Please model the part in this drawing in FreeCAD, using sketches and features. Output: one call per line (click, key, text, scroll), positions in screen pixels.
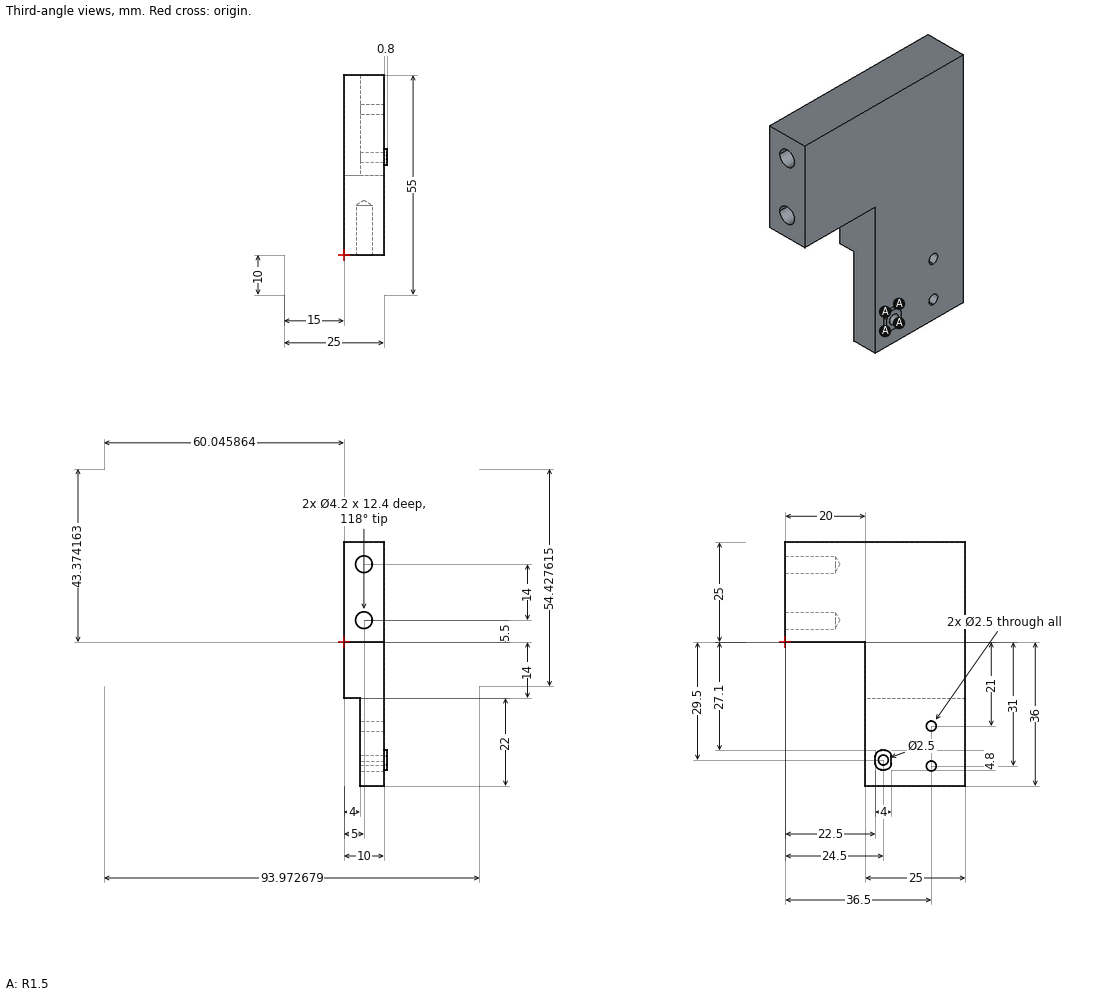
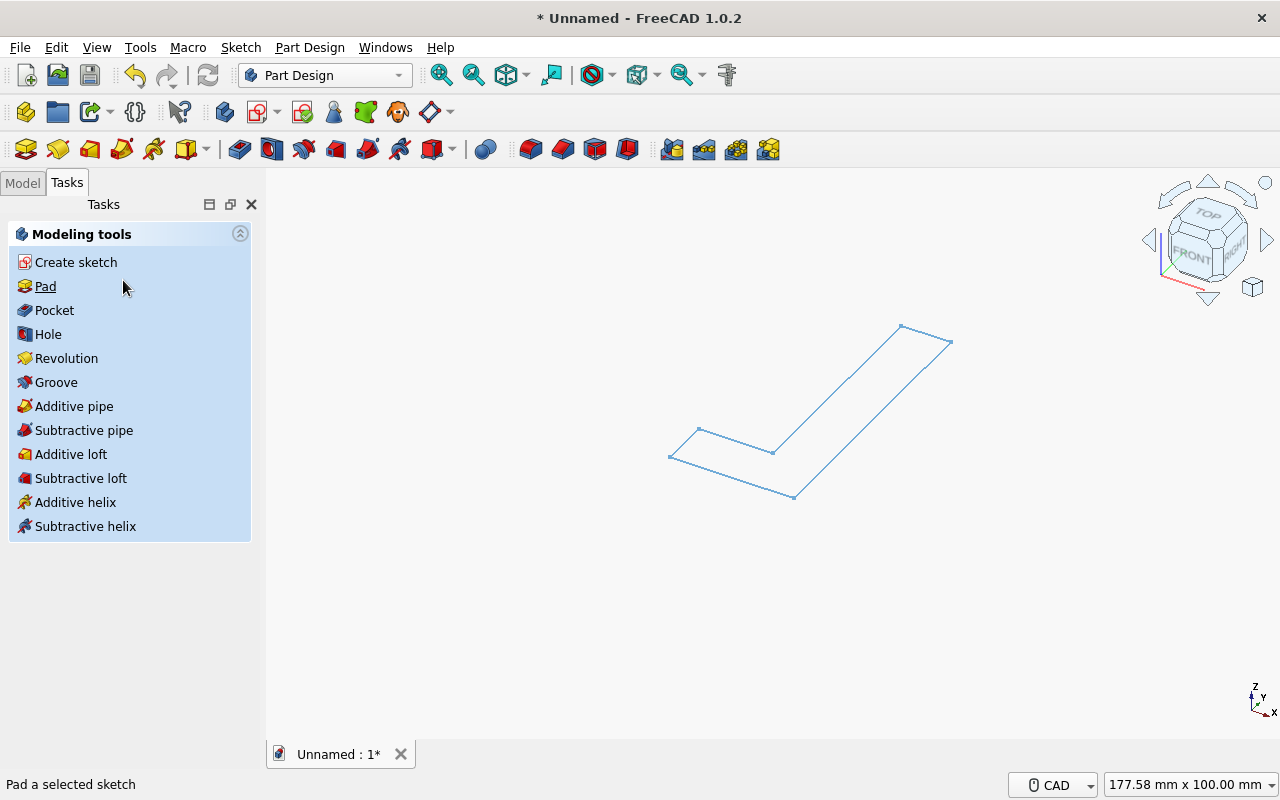
click(26, 150)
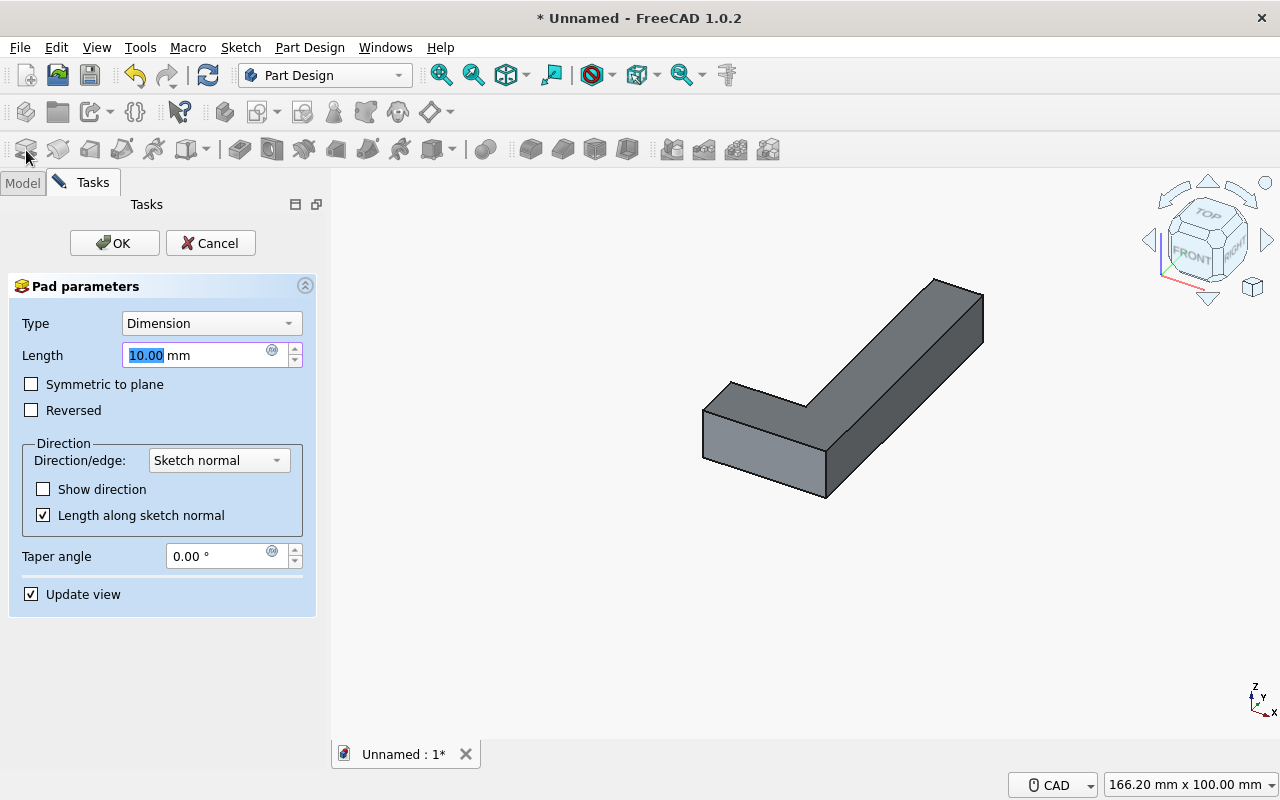
text(25)
key(Tab)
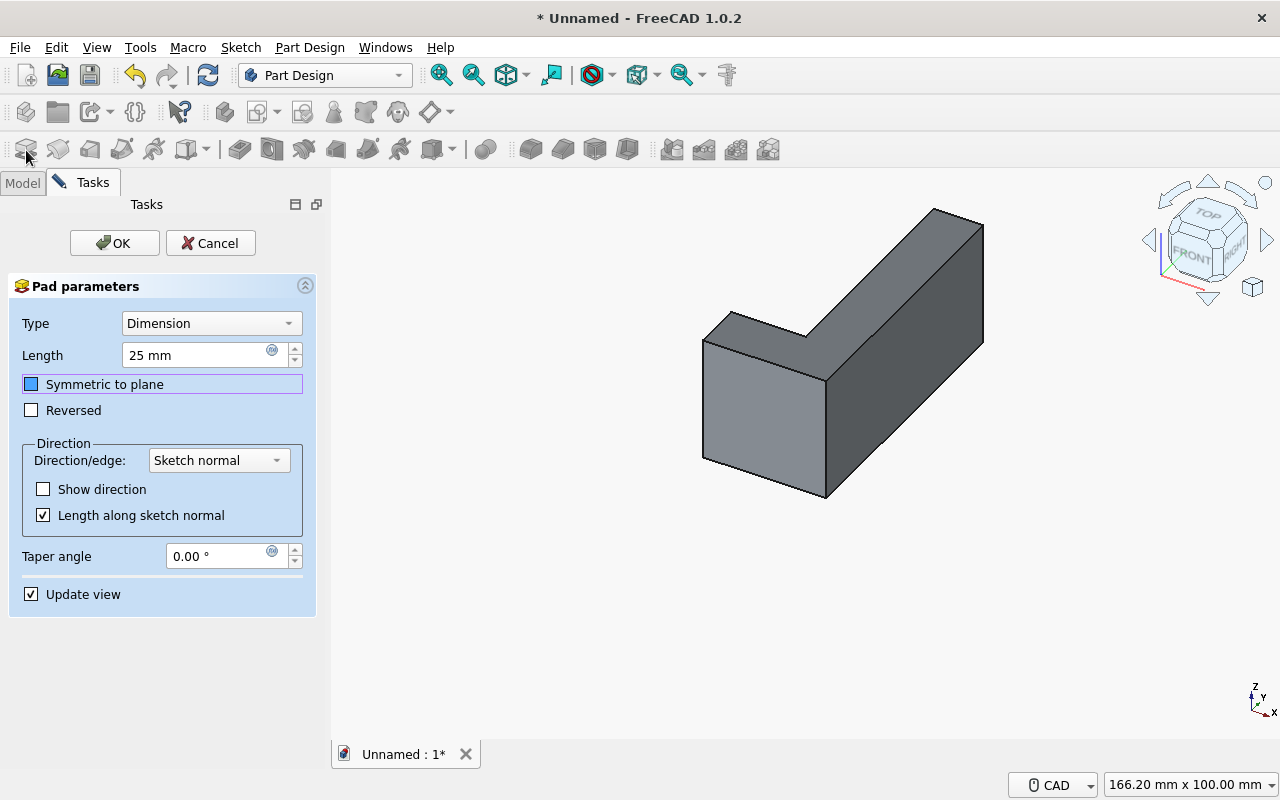
click(115, 243)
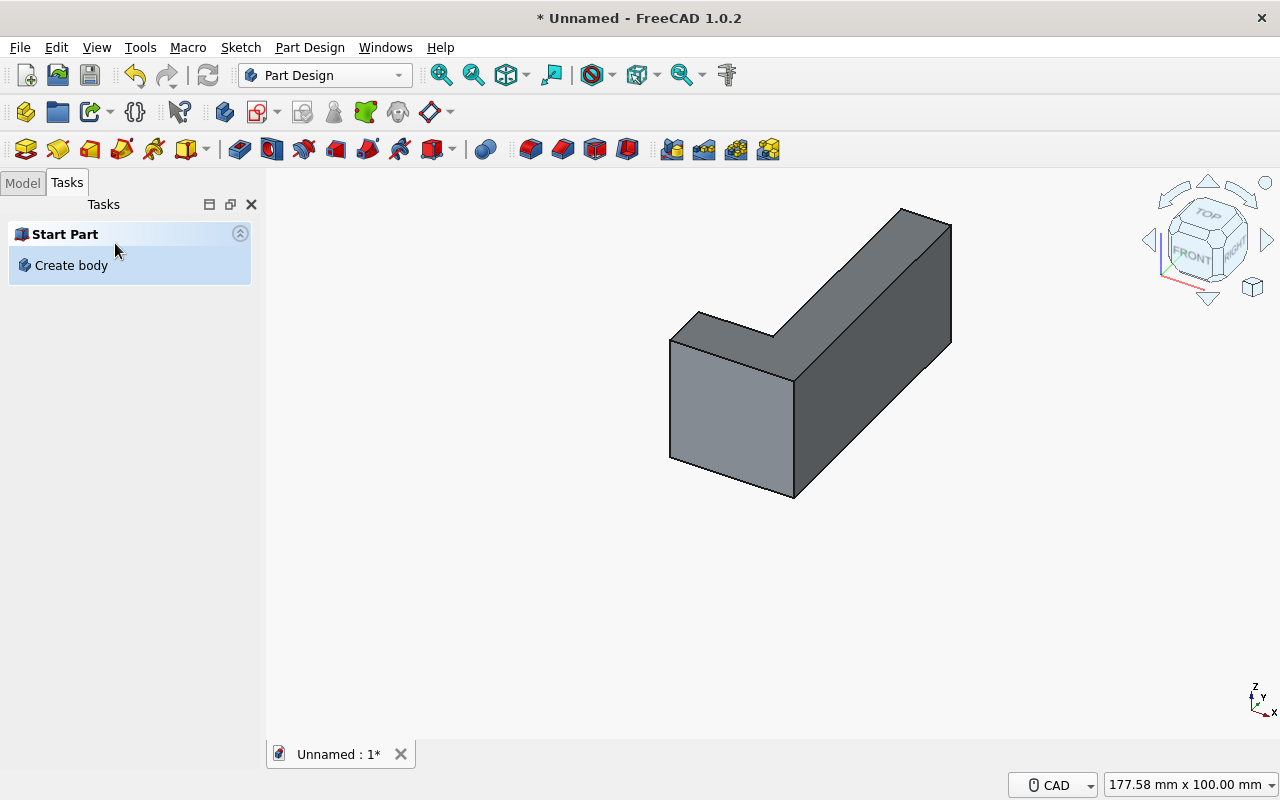
click(258, 112)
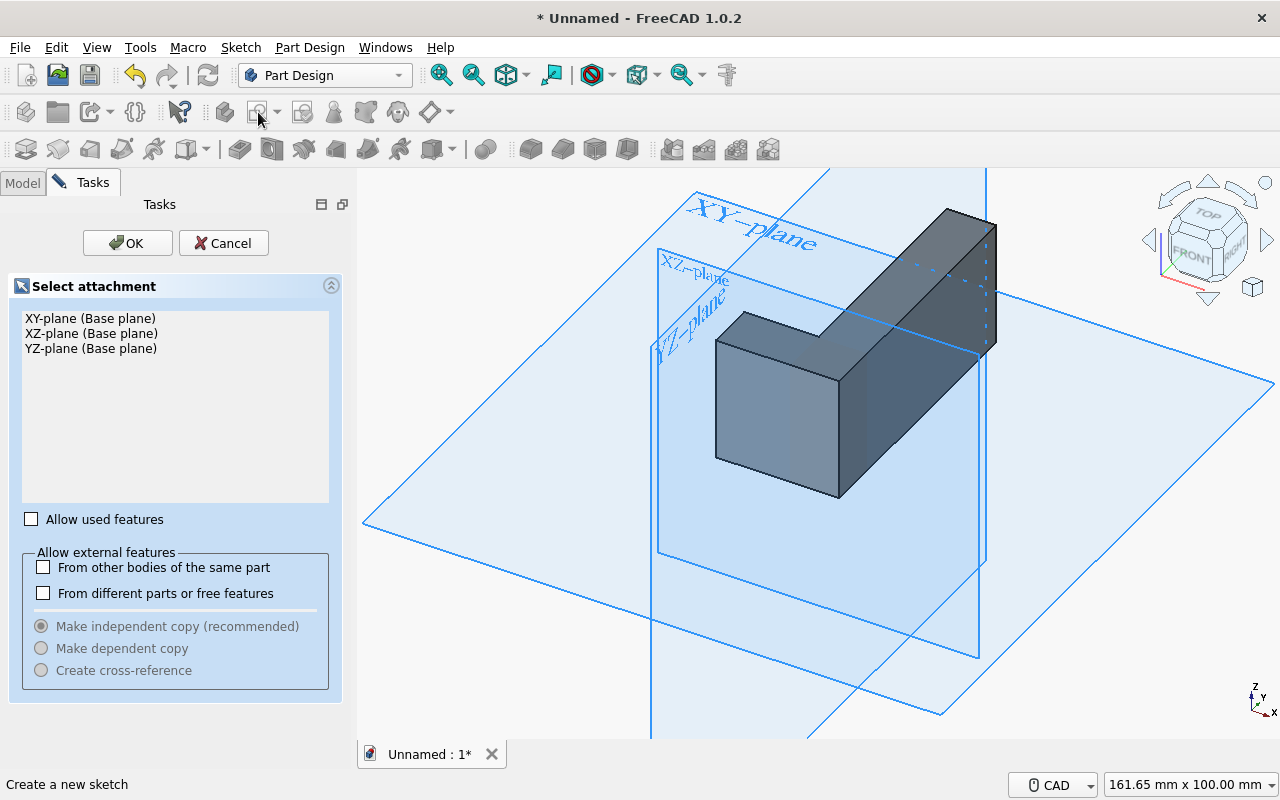
click(82, 348)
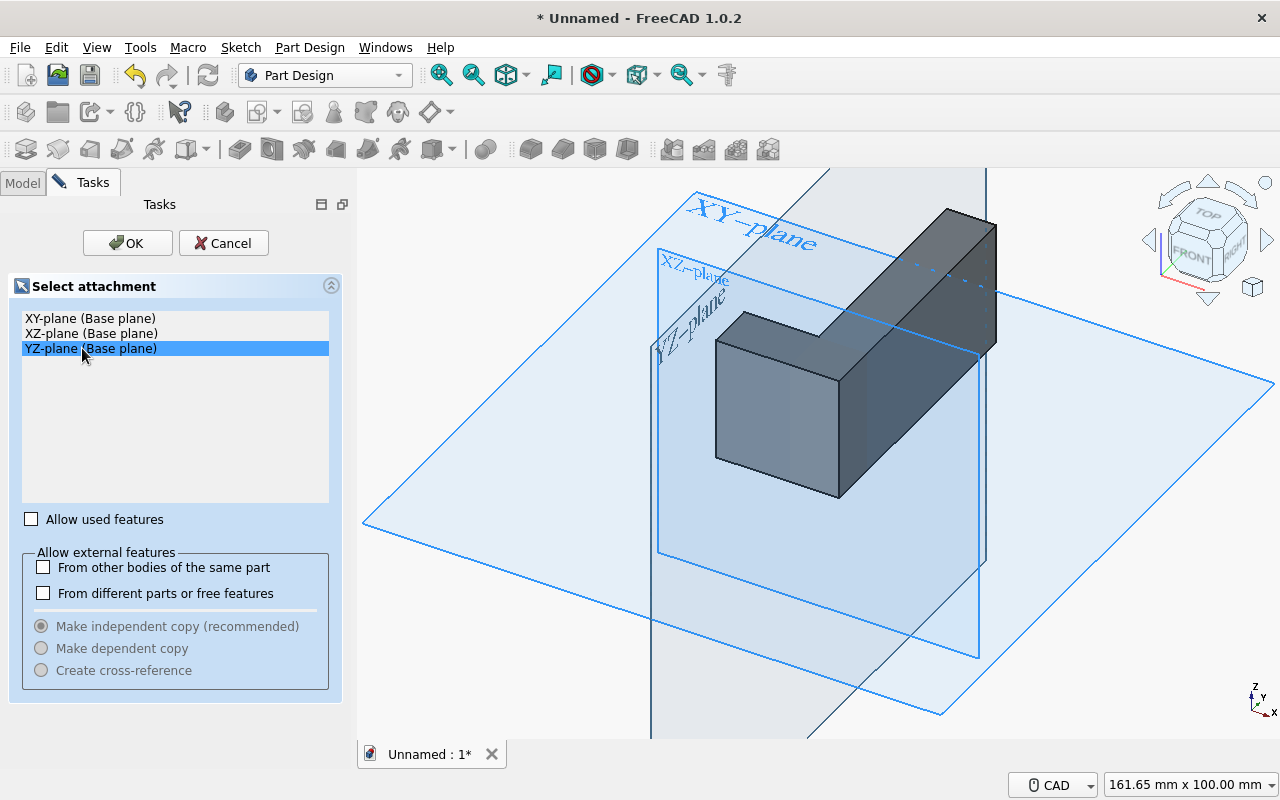
click(128, 243)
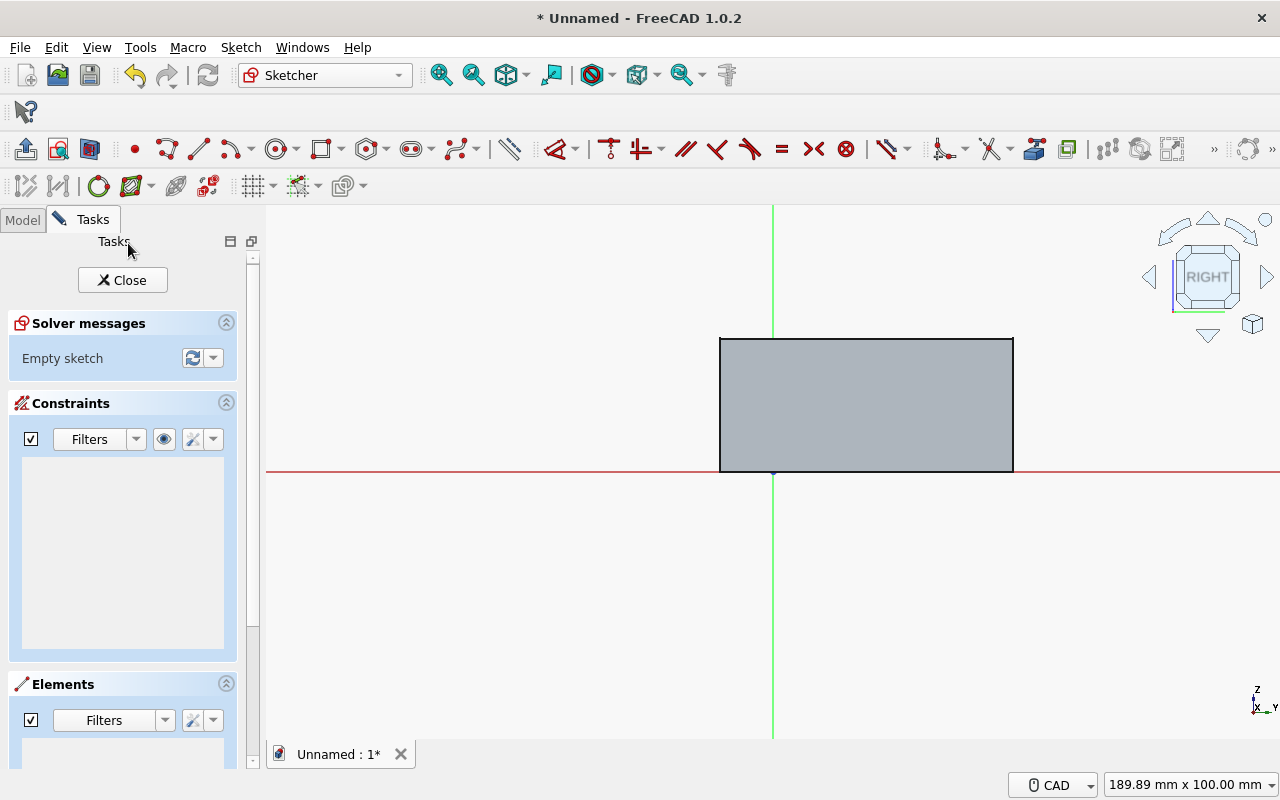
click(90, 150)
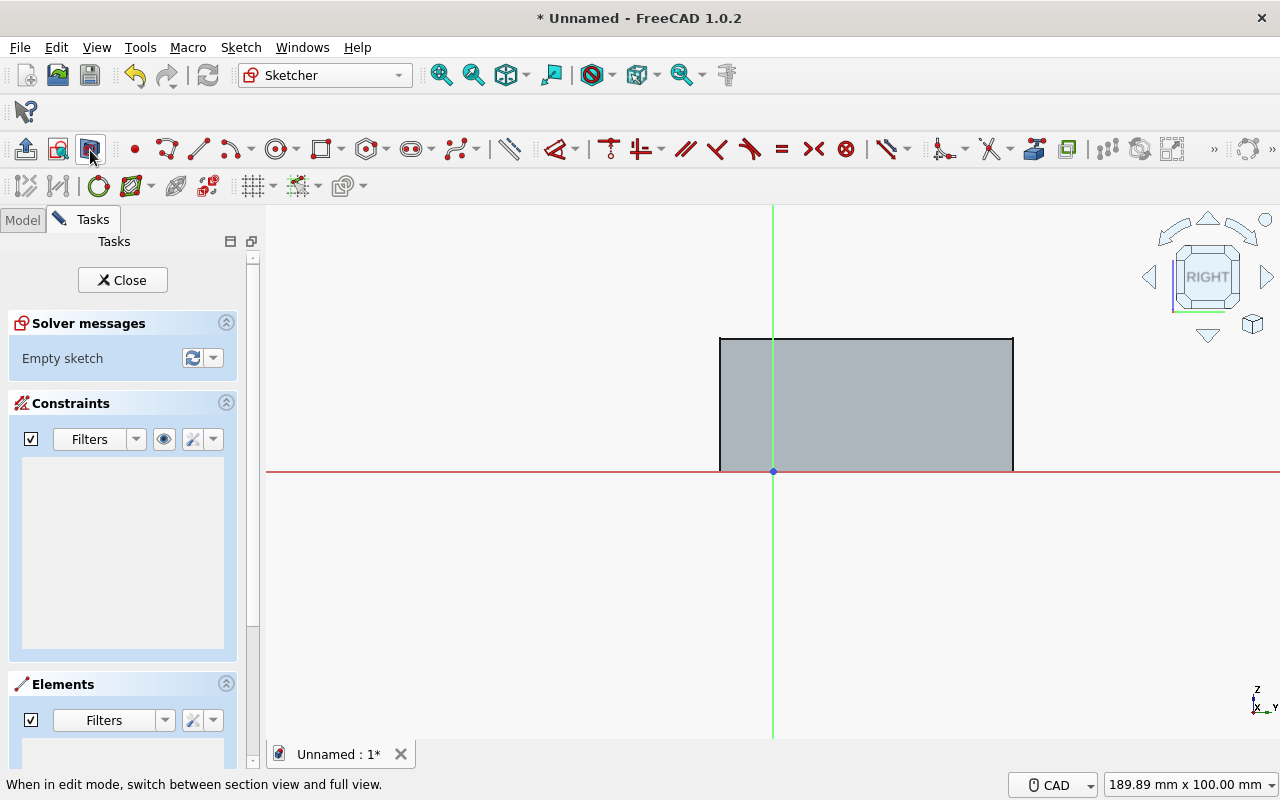
scroll(1115, 685, up, 3)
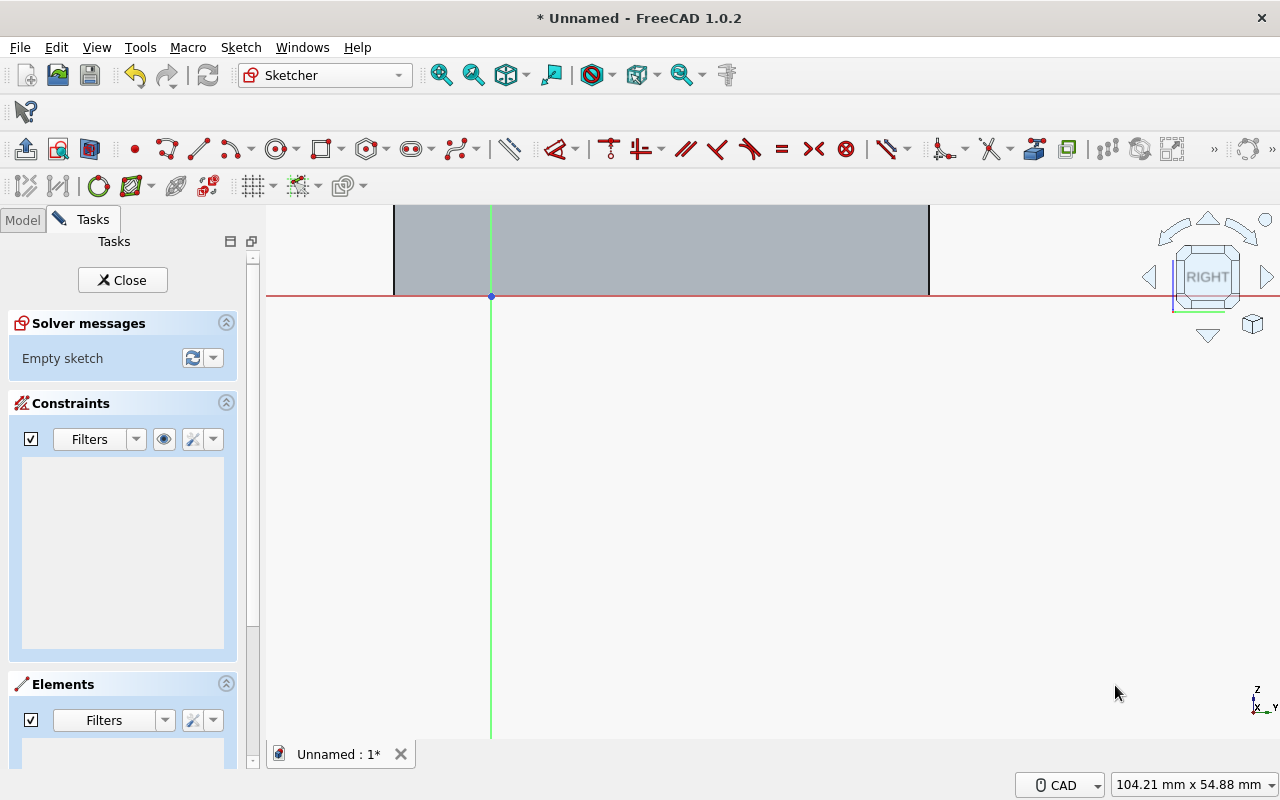
click(322, 150)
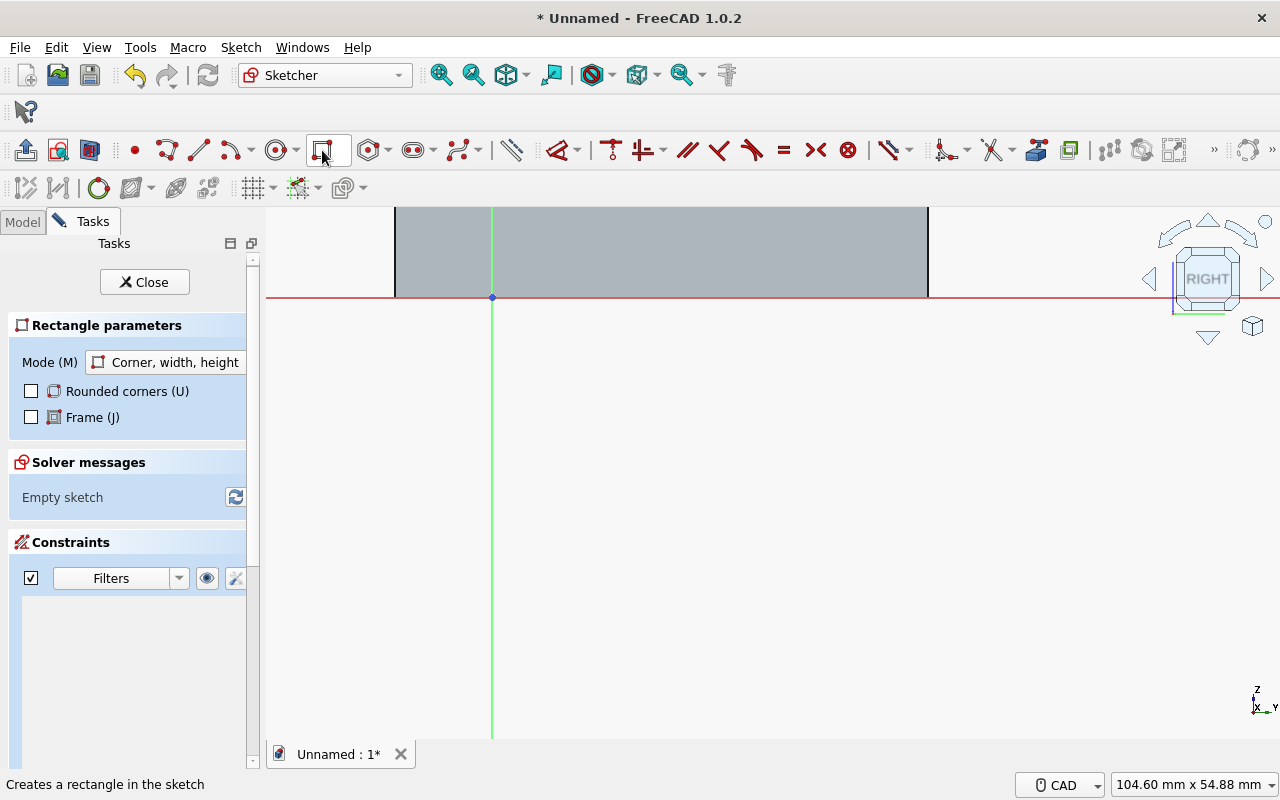
click(686, 298)
move(928, 647)